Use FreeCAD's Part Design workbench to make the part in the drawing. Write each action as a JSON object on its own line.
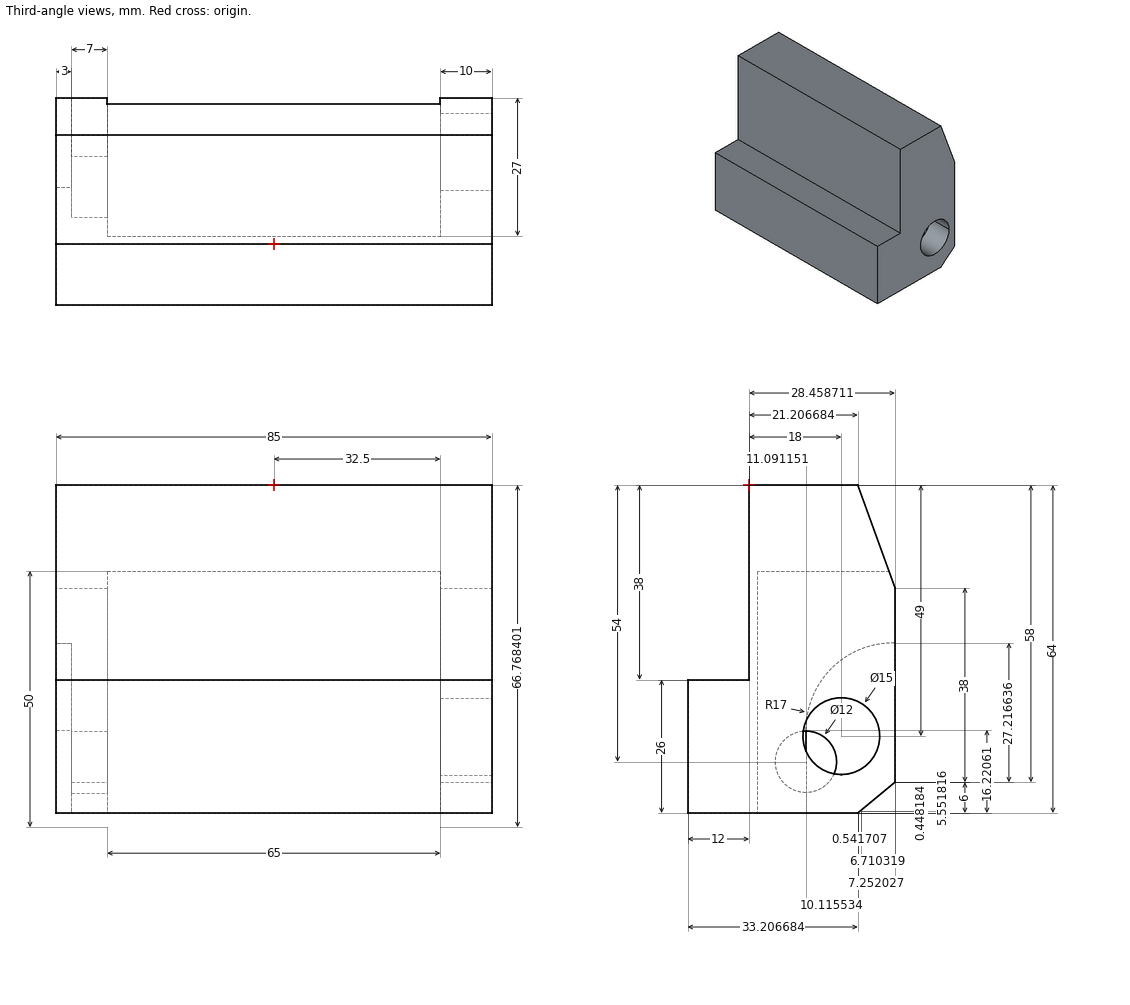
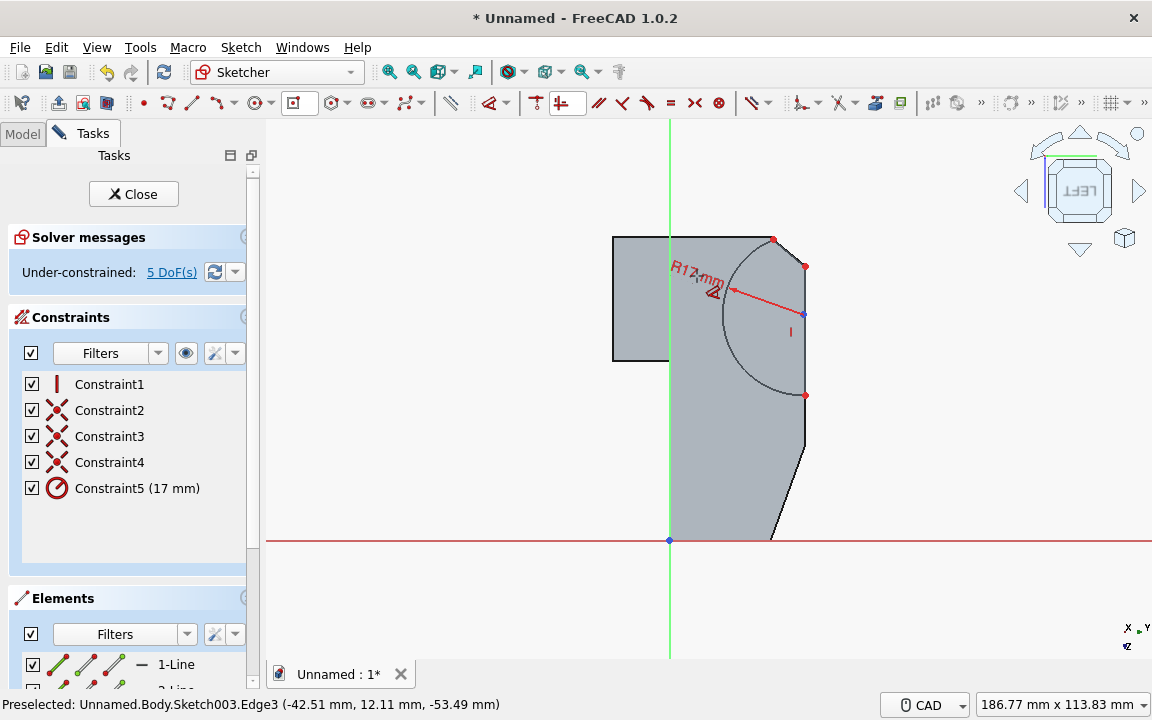
{"action": "left_click", "coordinate": [805, 267]}
{"action": "left_click", "coordinate": [839, 404]}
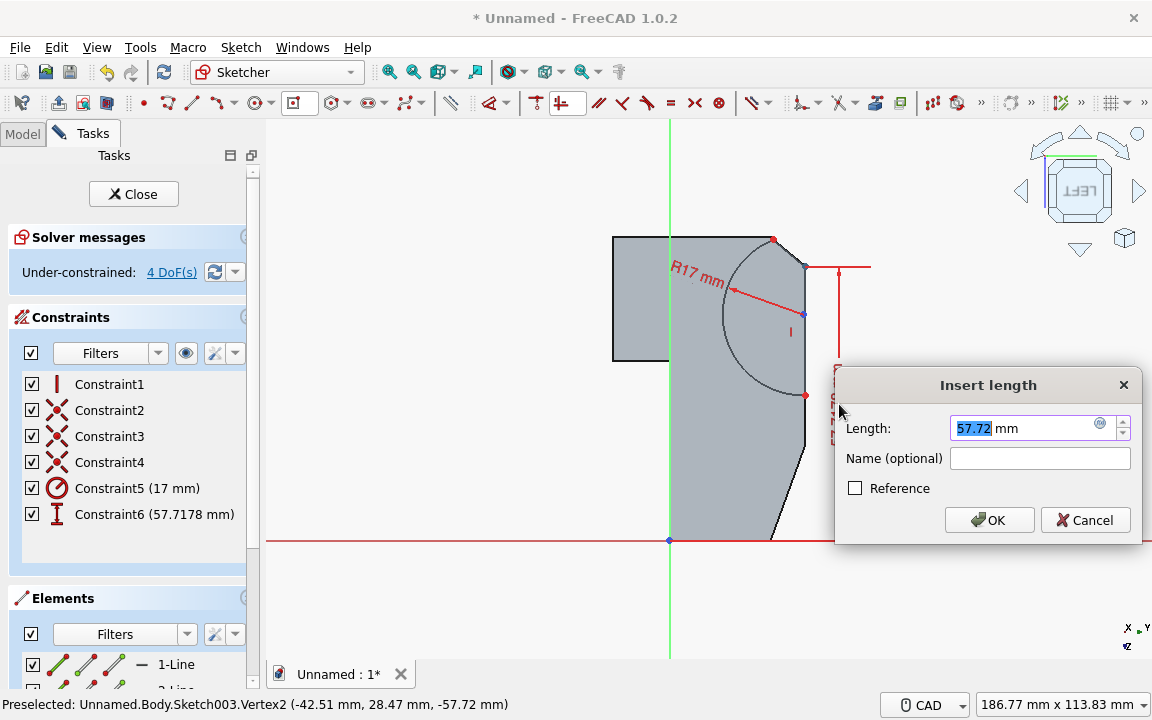
{"action": "type", "text": "58"}
{"action": "key", "text": "Return"}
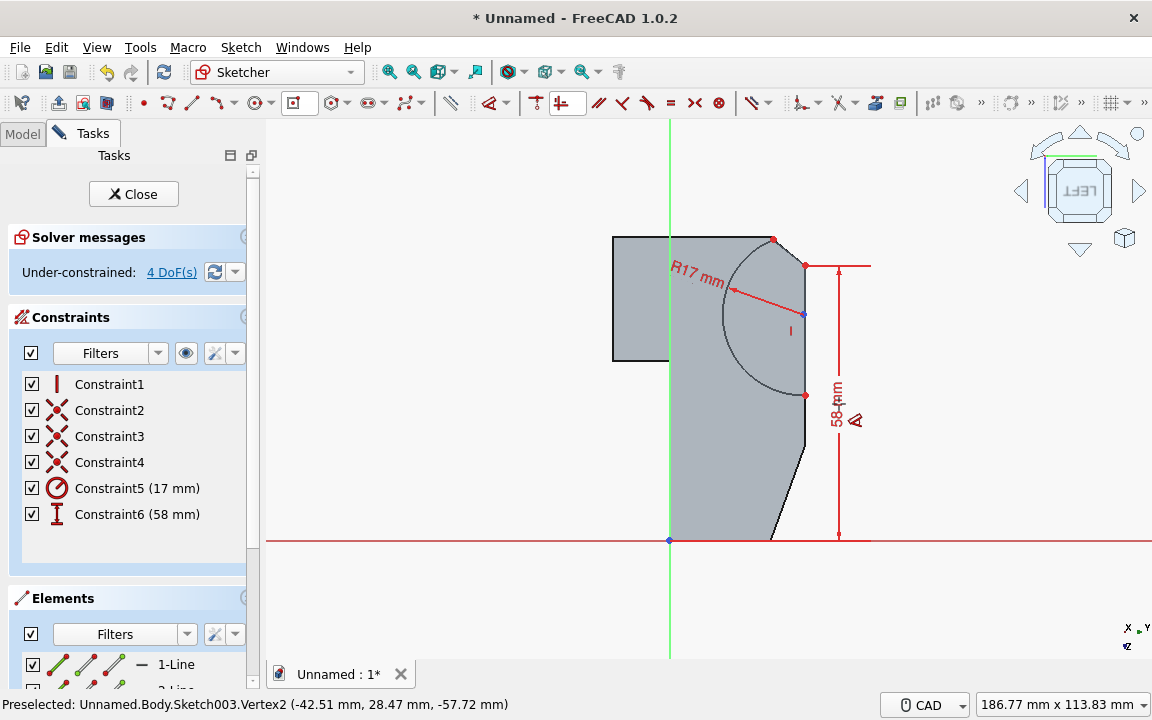
{"action": "left_click", "coordinate": [805, 356]}
{"action": "left_click", "coordinate": [839, 330]}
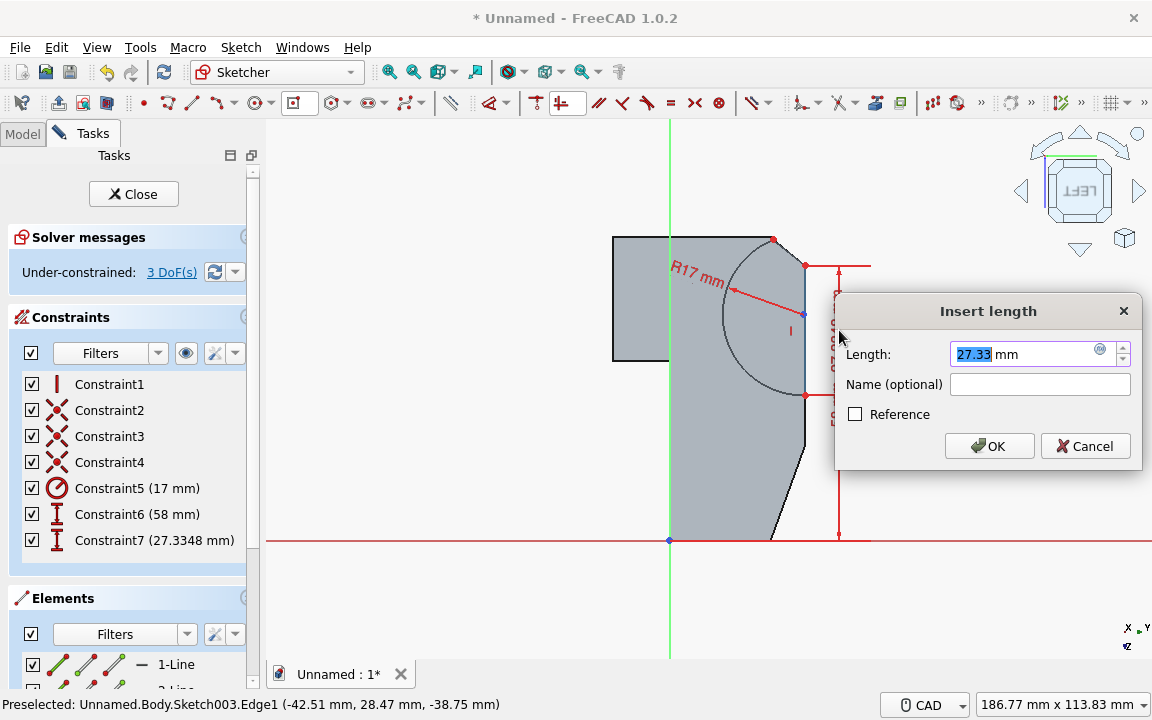
{"action": "type", "text": "27.216636"}
{"action": "key", "text": "Return"}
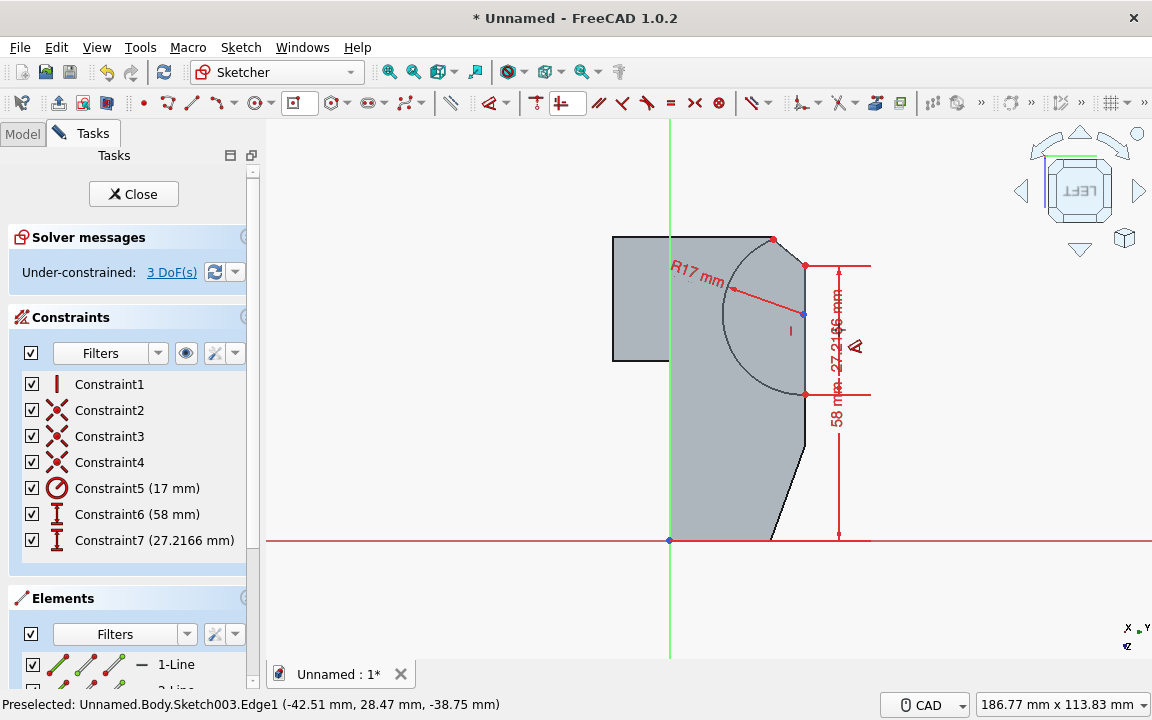
{"action": "scroll", "coordinate": [795, 258], "scroll_direction": "up", "scroll_amount": 2}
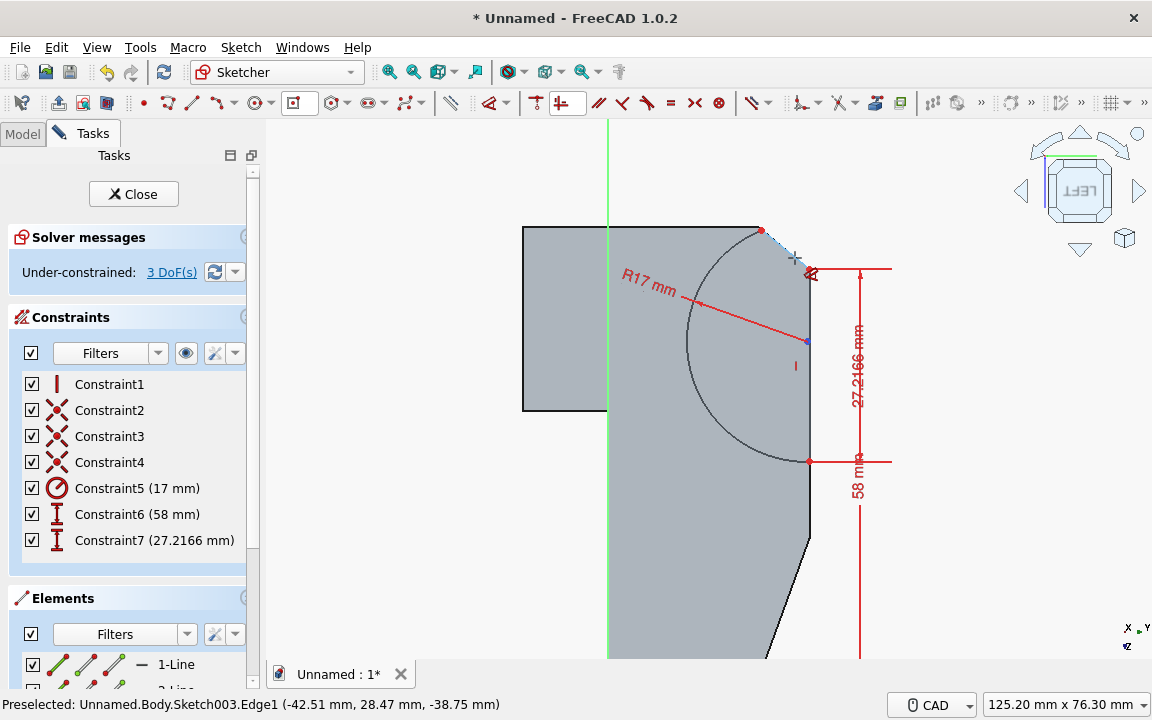
{"action": "left_click", "coordinate": [795, 258]}
{"action": "left_click", "coordinate": [786, 196]}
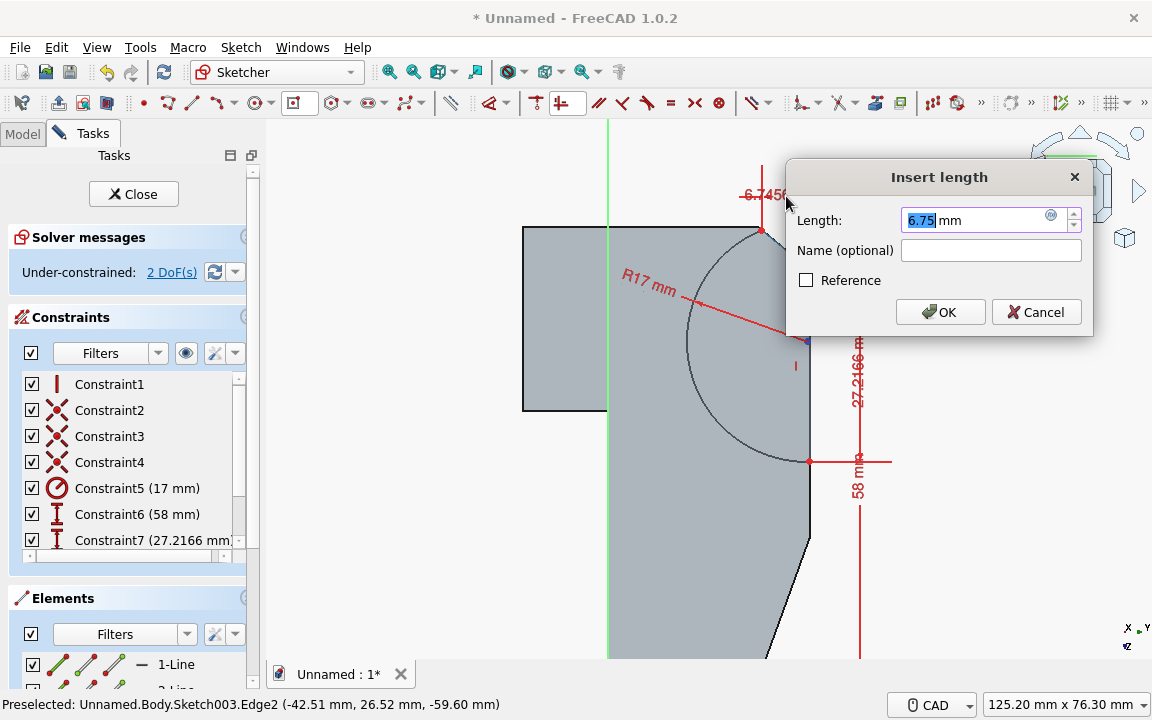
{"action": "type", "text": "6.710319"}
{"action": "key", "text": "Return"}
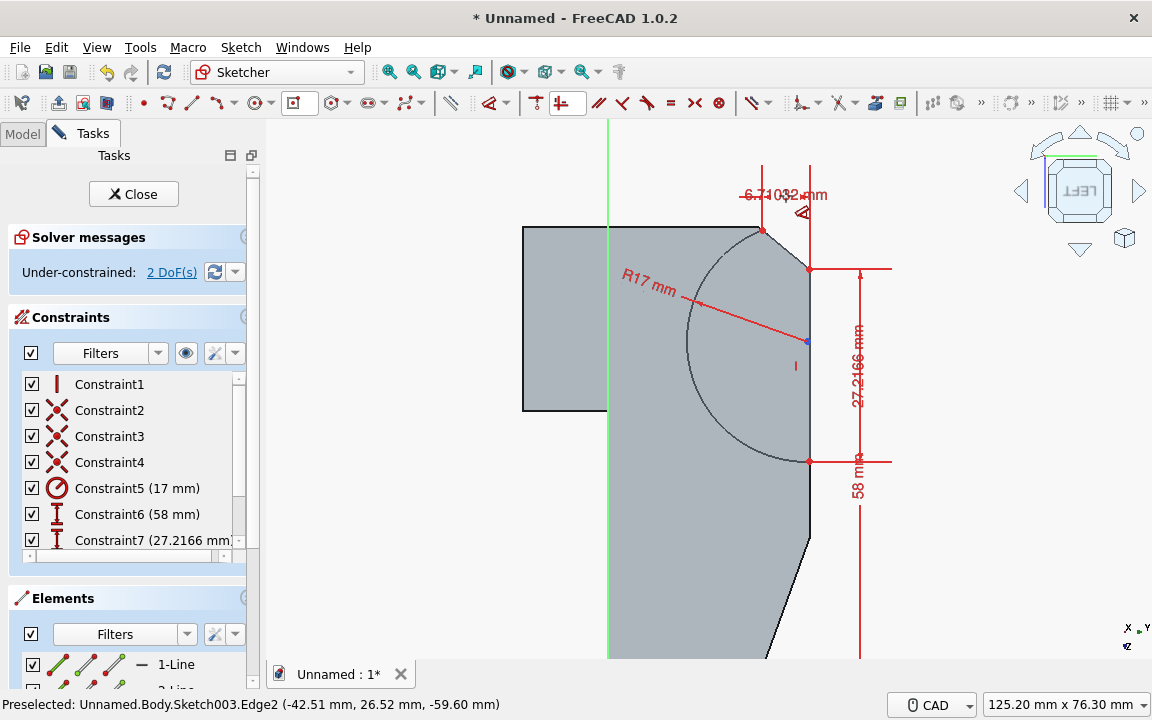
{"action": "left_click", "coordinate": [795, 258]}
{"action": "left_click", "coordinate": [844, 250]}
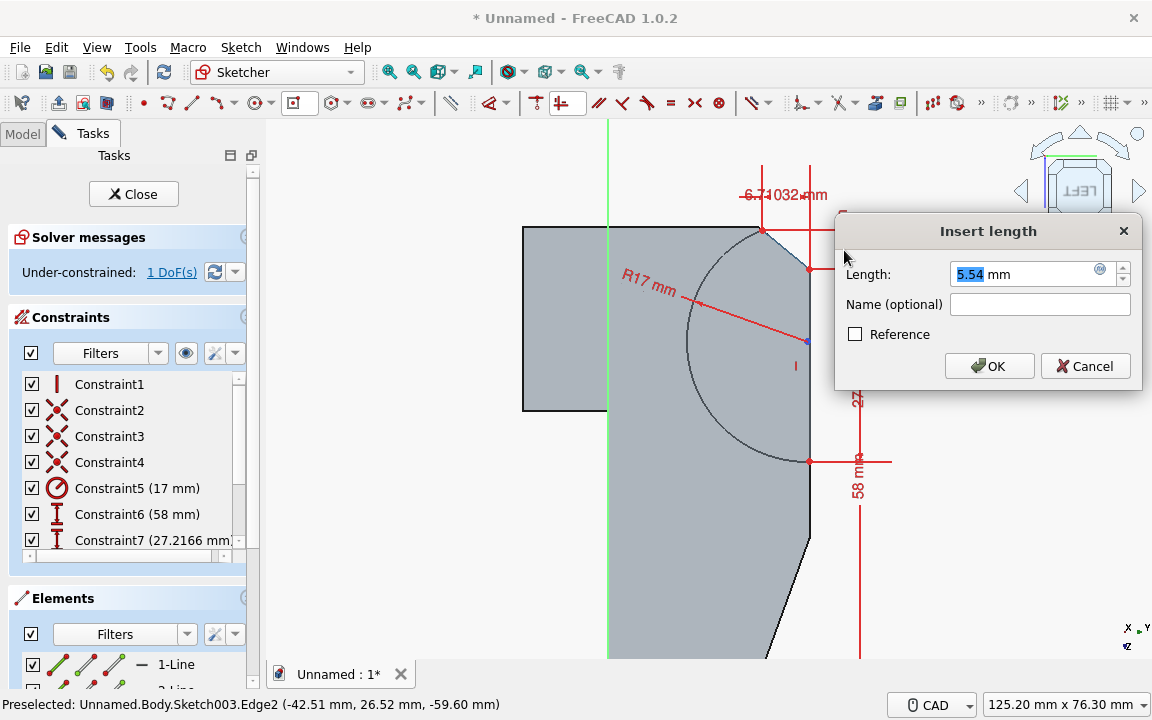
{"action": "type", "text": "5.551816"}
{"action": "key", "text": "Return"}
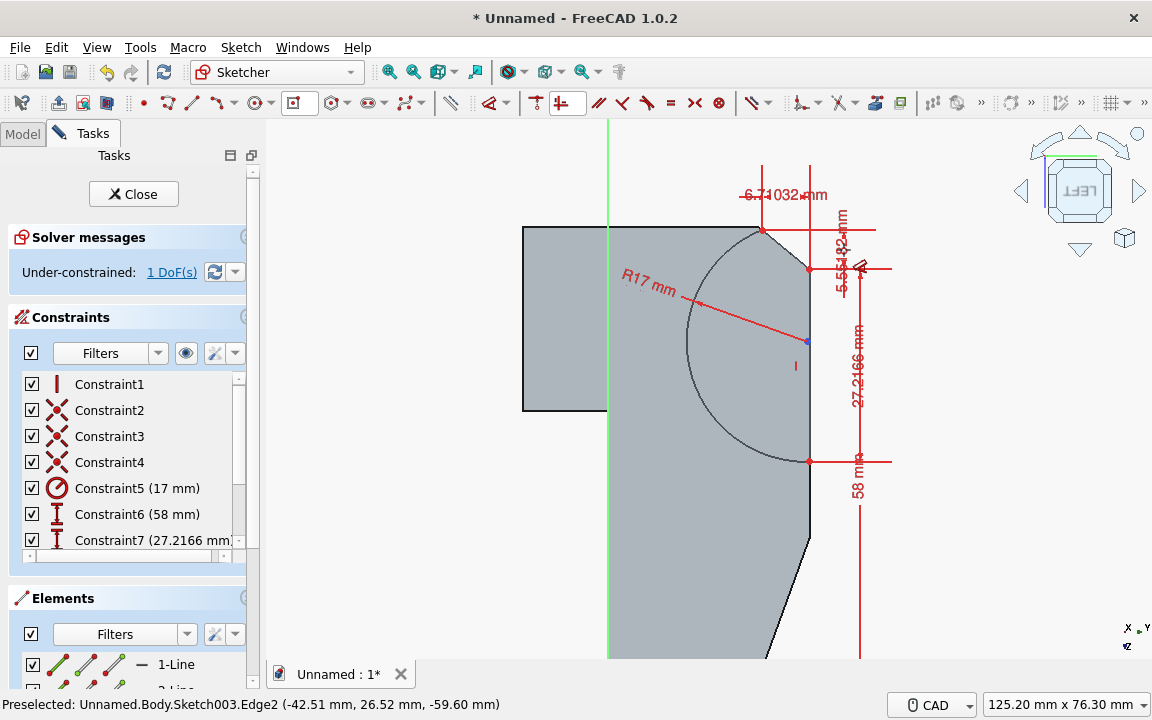
{"action": "left_click", "coordinate": [810, 462]}
{"action": "left_click", "coordinate": [663, 428]}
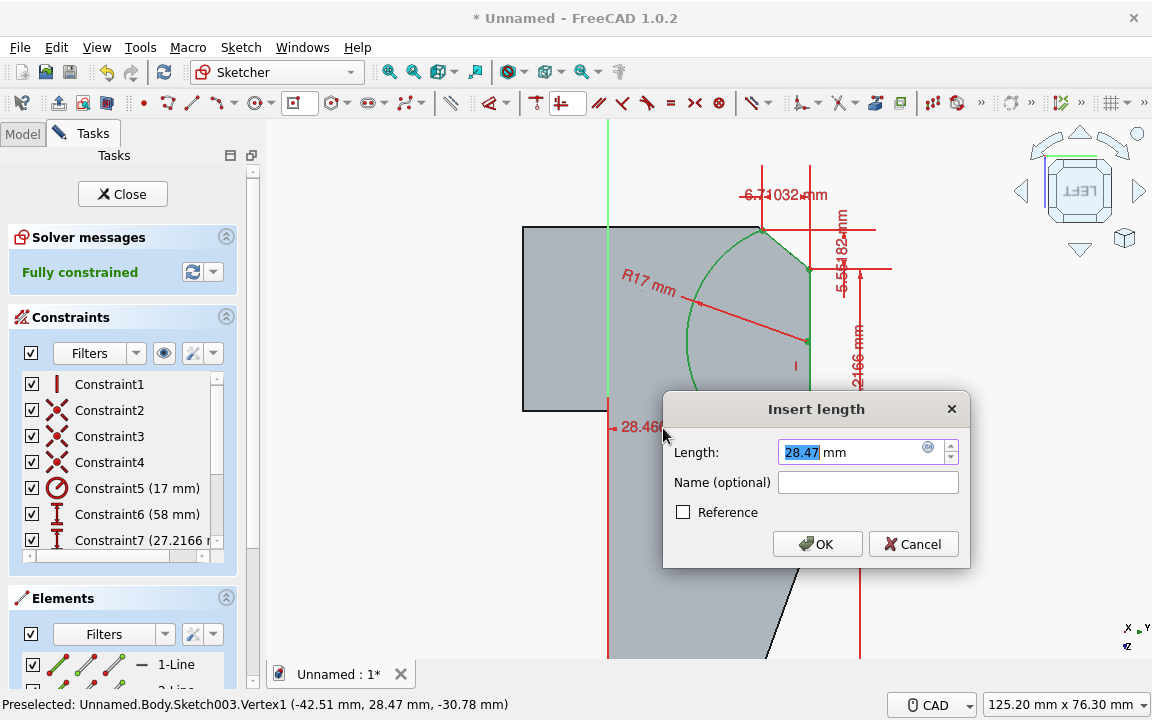
{"action": "type", "text": "28.458711"}
{"action": "key", "text": "Return"}
{"action": "key", "text": "Escape"}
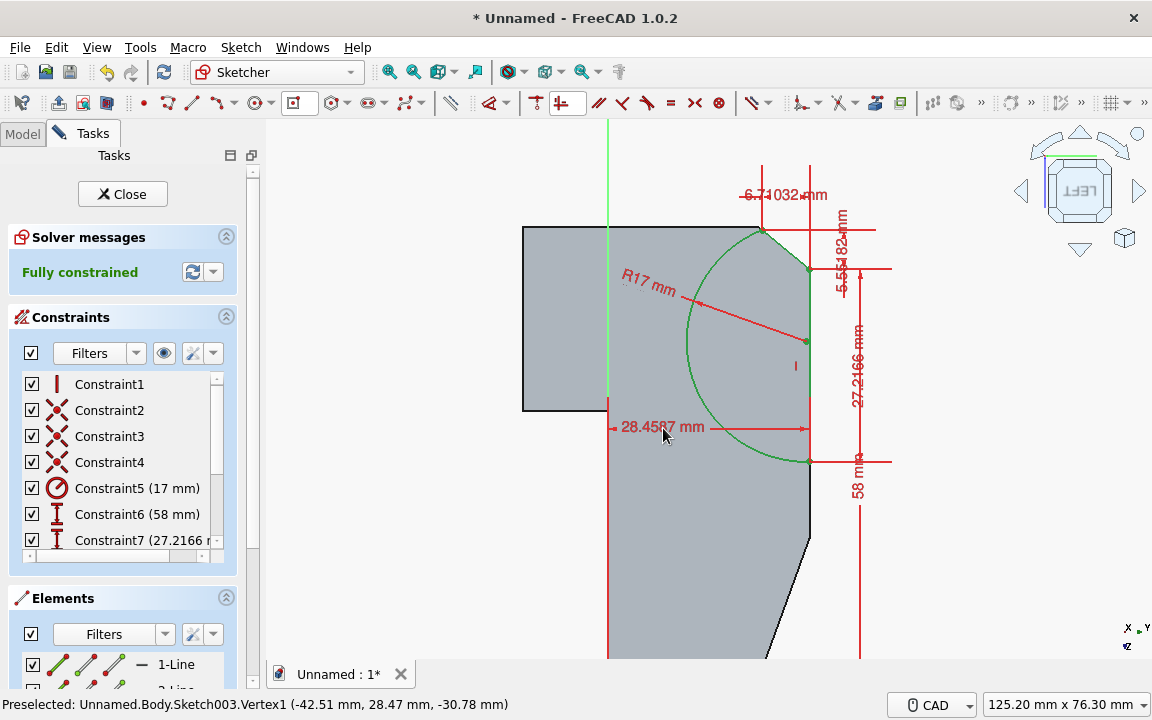
{"action": "left_click", "coordinate": [123, 194]}